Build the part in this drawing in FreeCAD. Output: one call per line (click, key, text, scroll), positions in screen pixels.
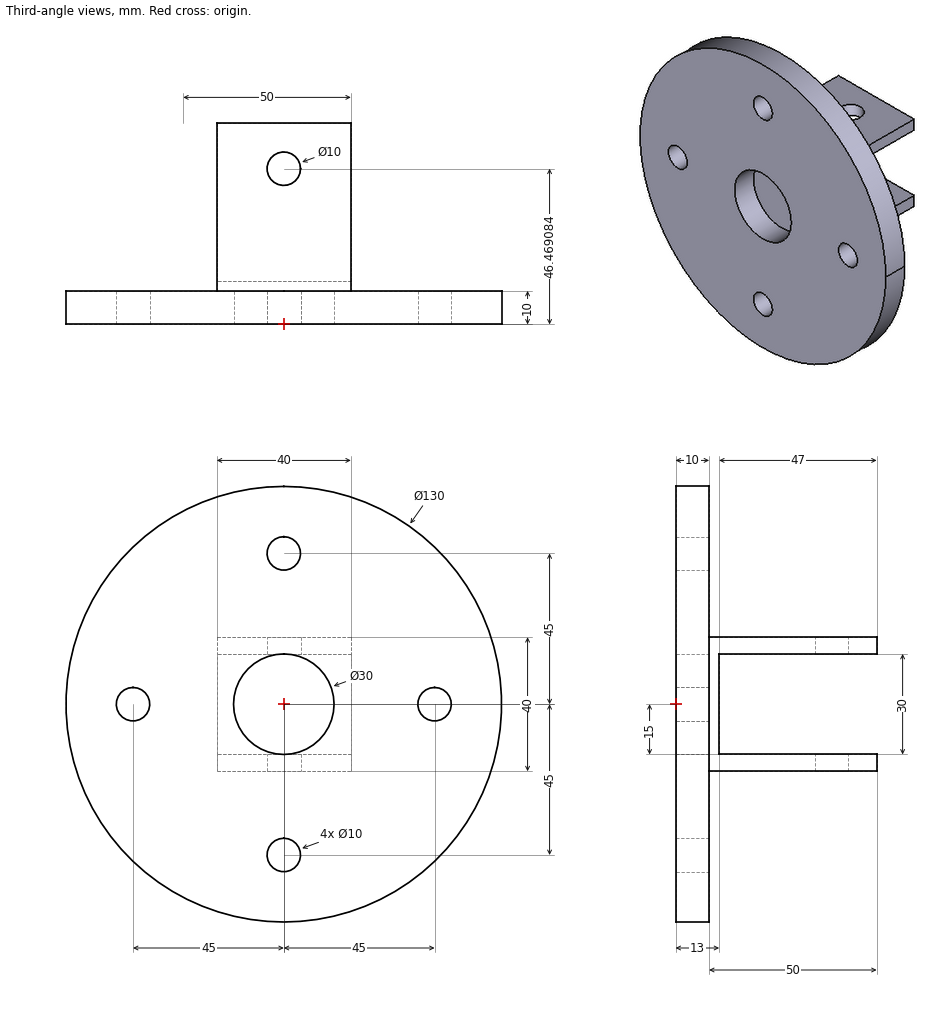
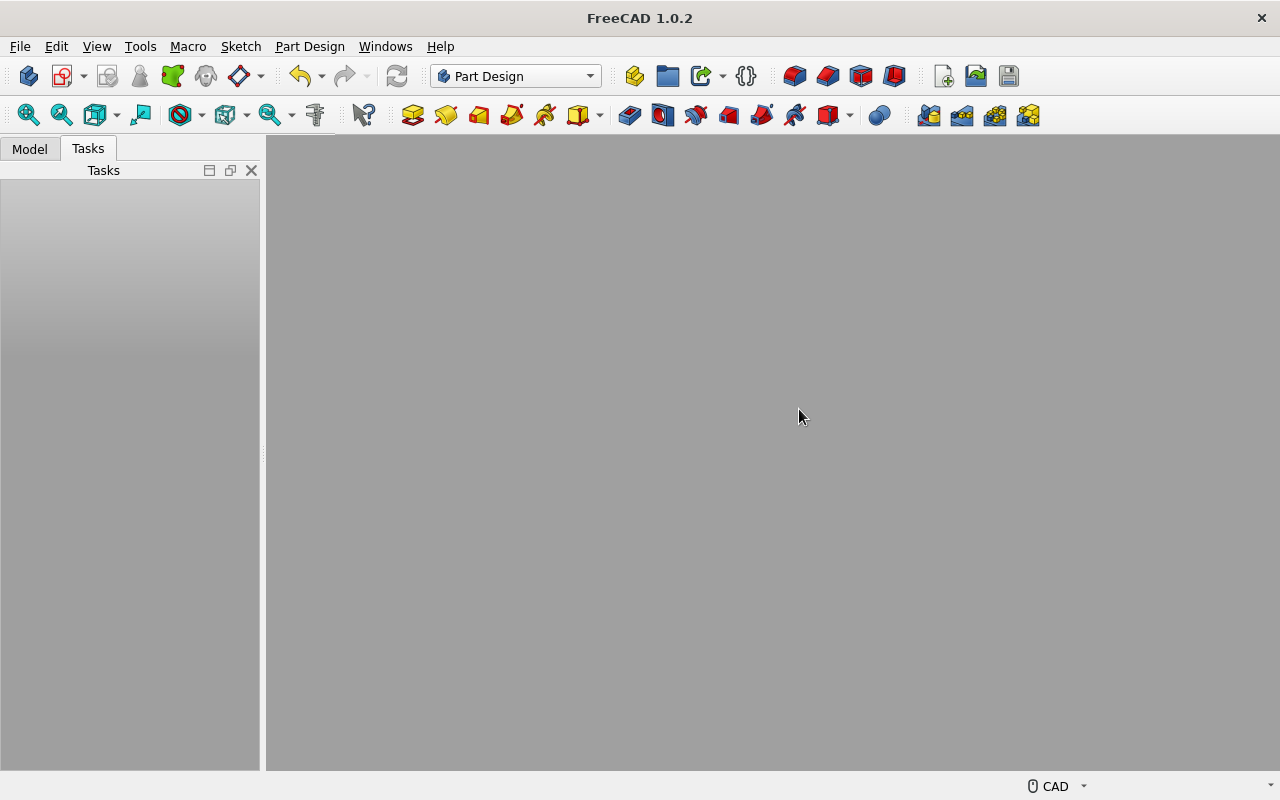
click(943, 76)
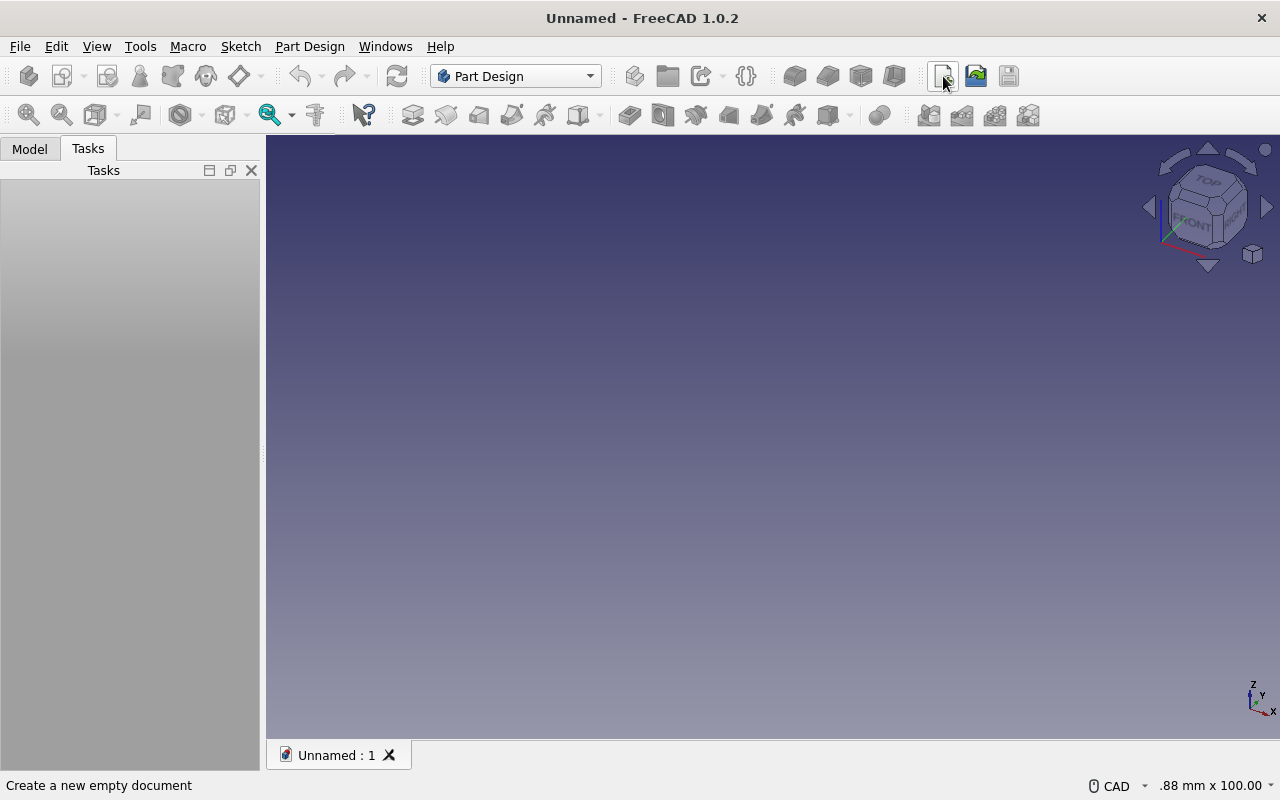
click(62, 76)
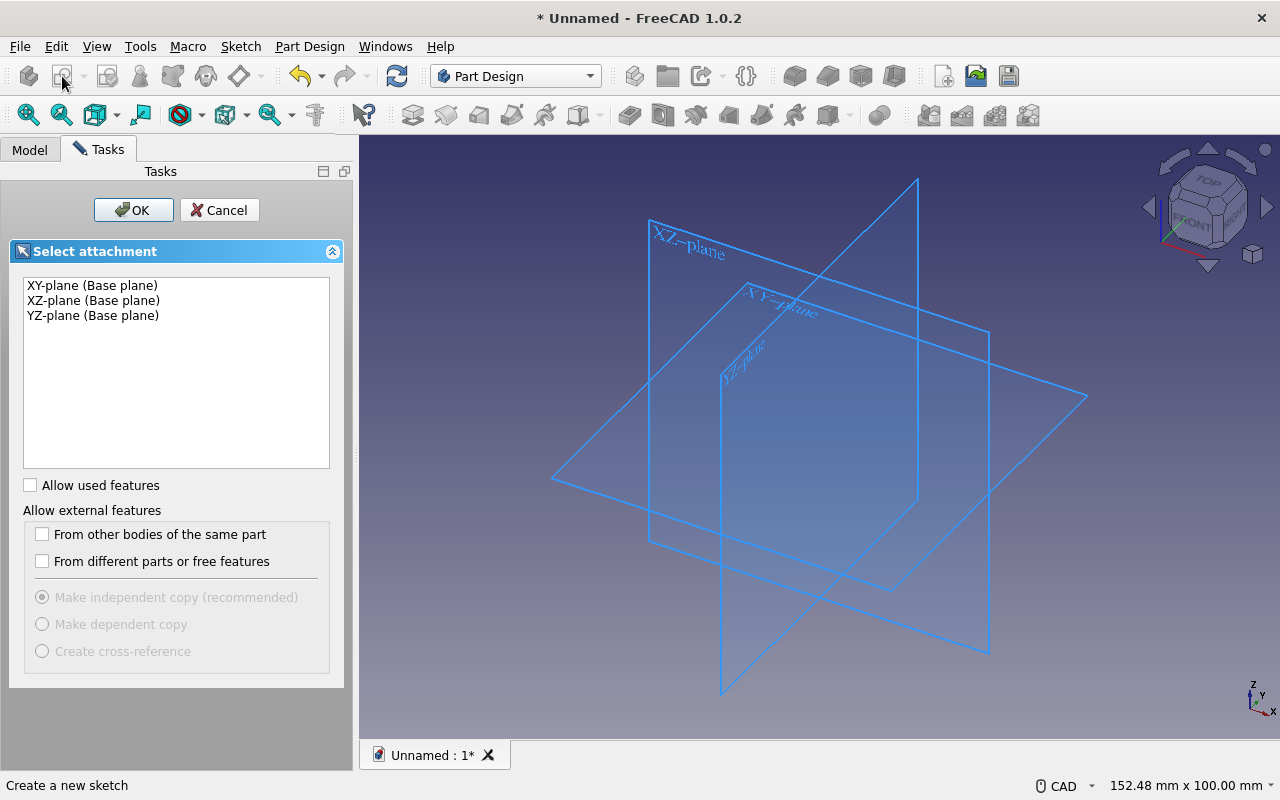
click(84, 300)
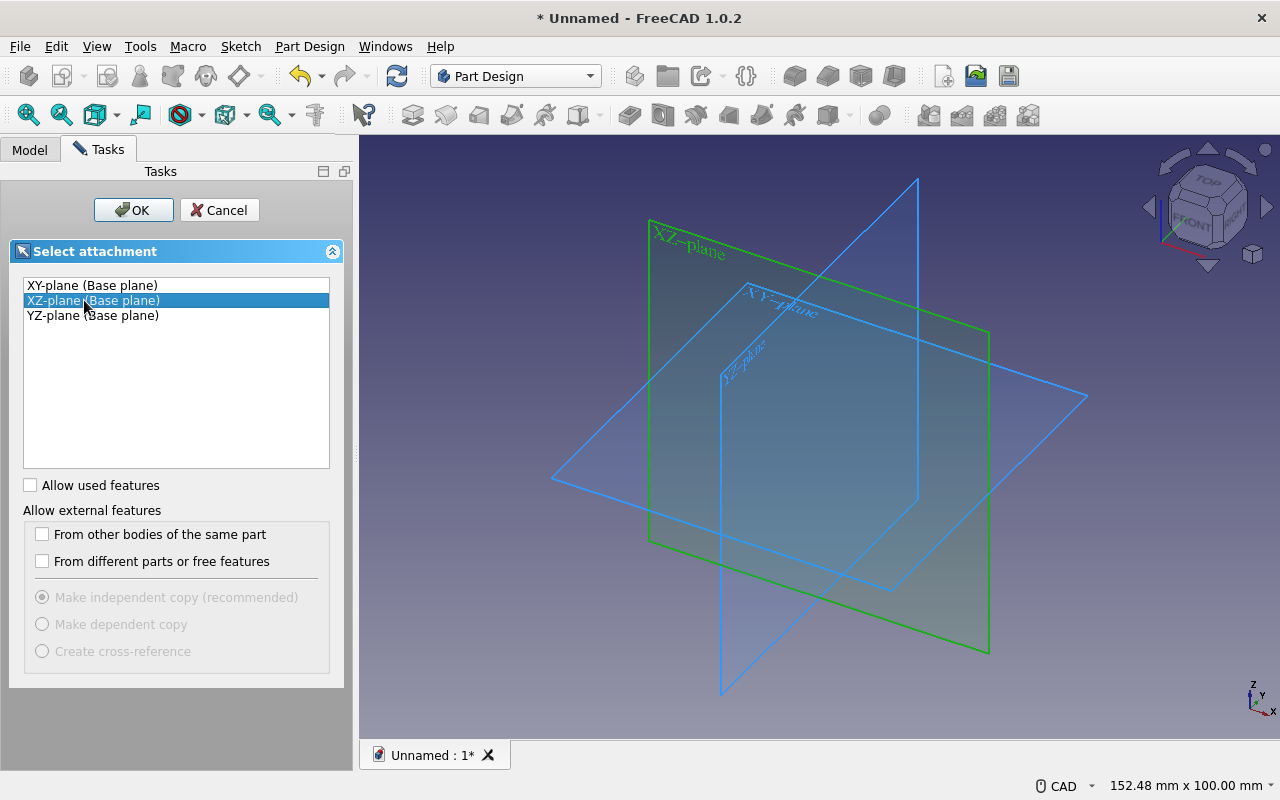
click(134, 210)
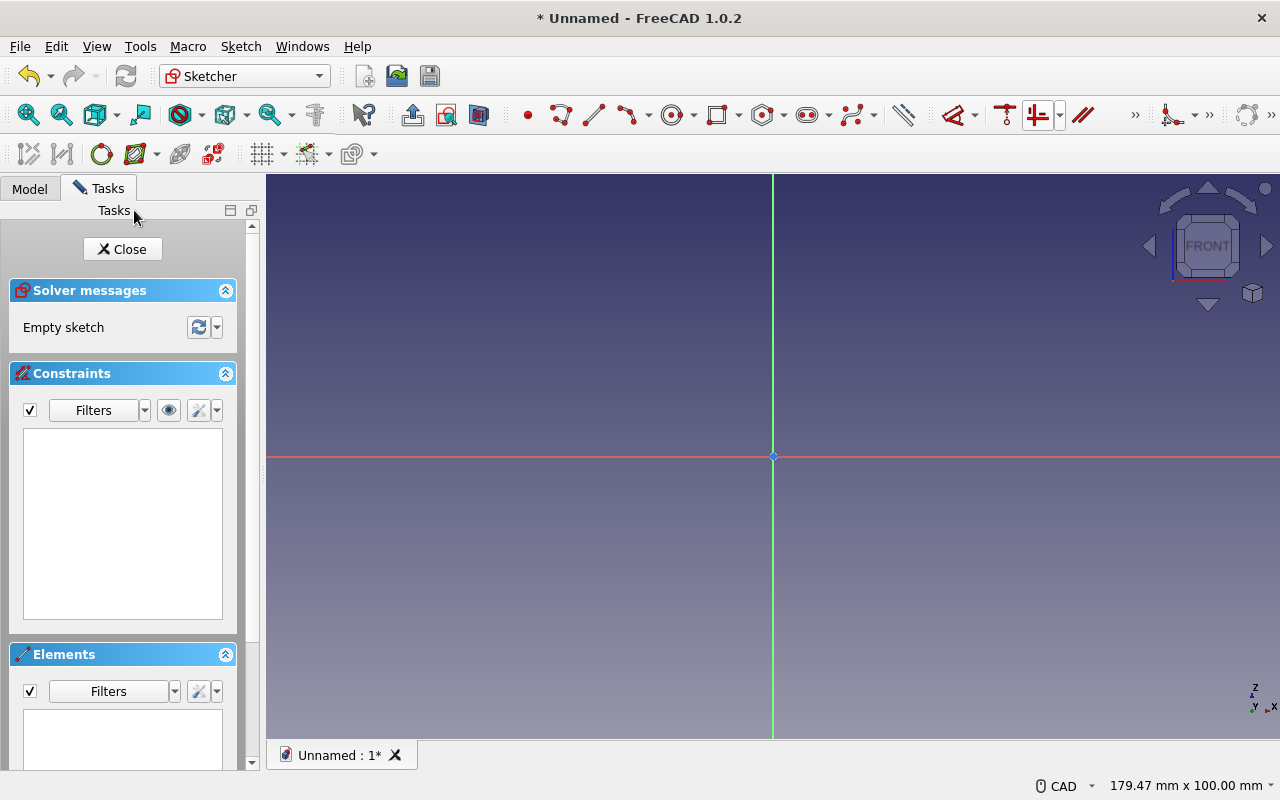
scroll(649, 456, down, 4)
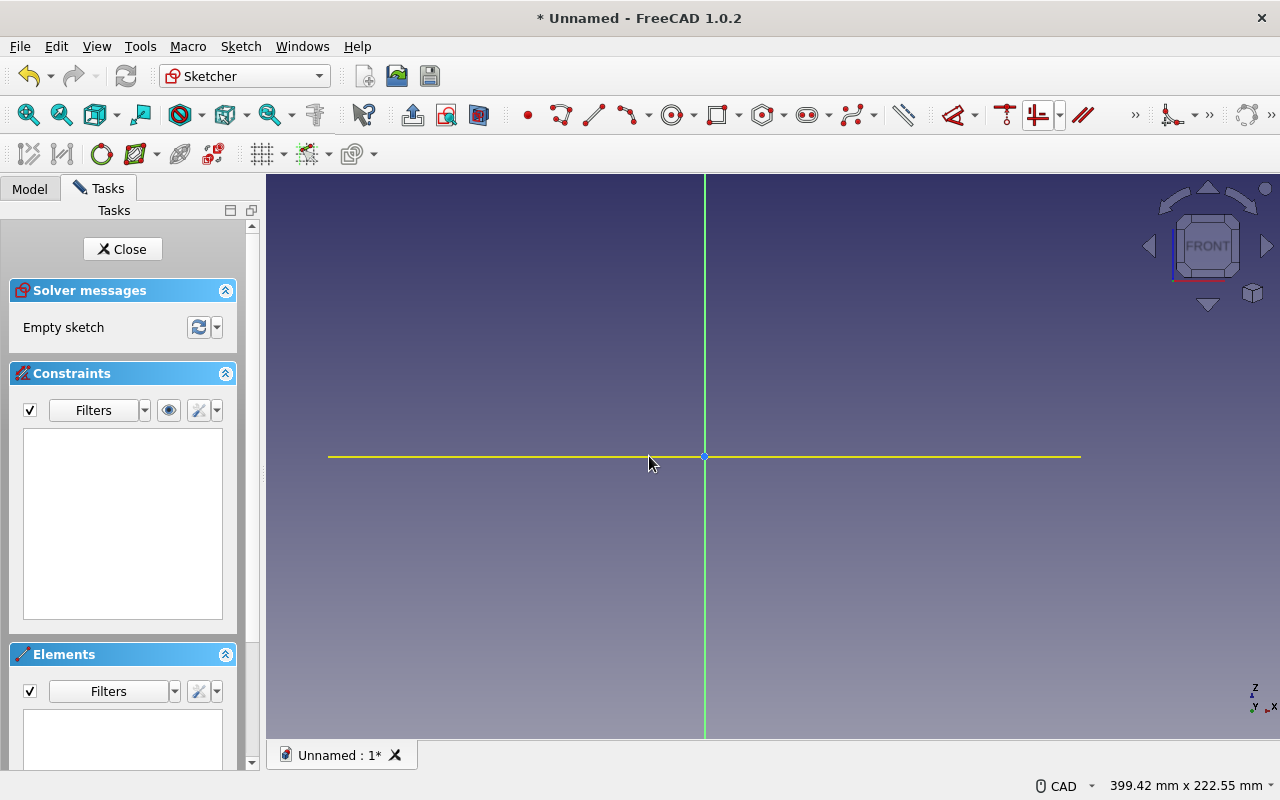
key(g)
key(c)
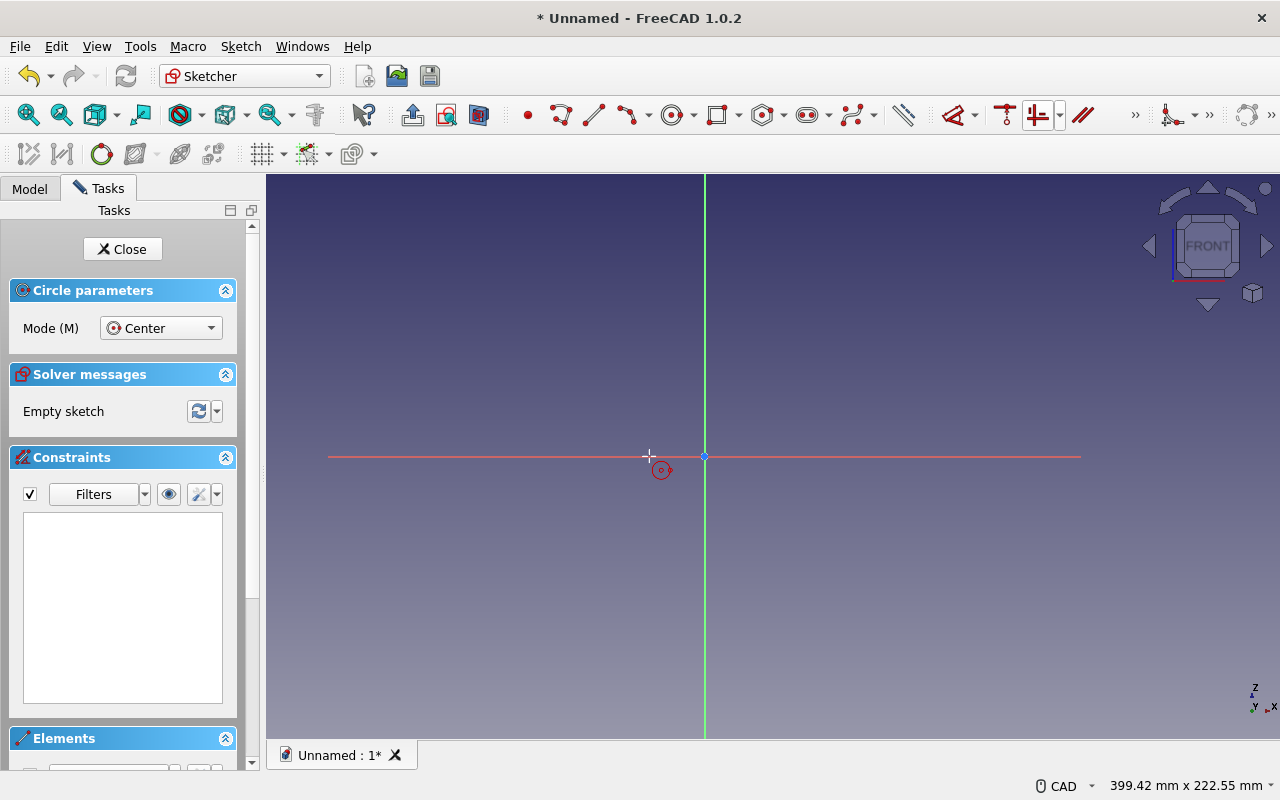
click(705, 456)
move(822, 340)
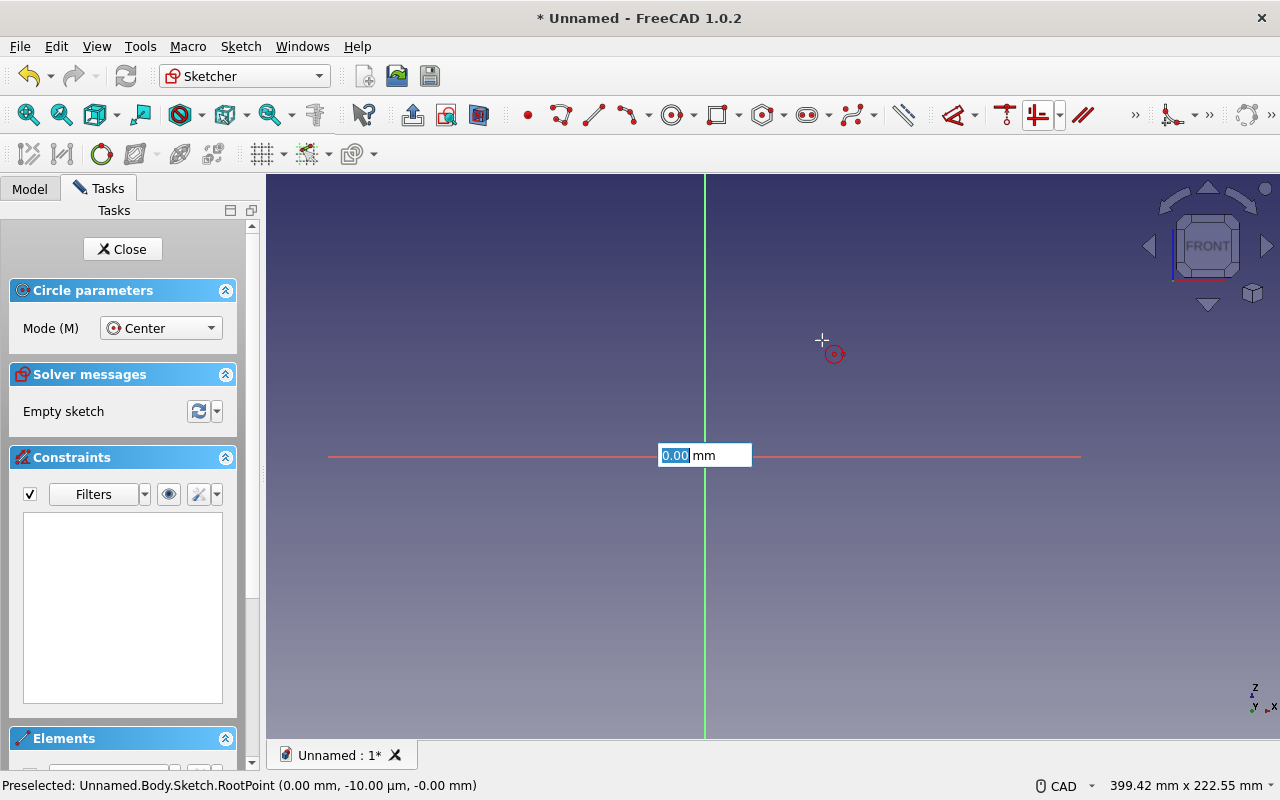
text(130)
key(Return)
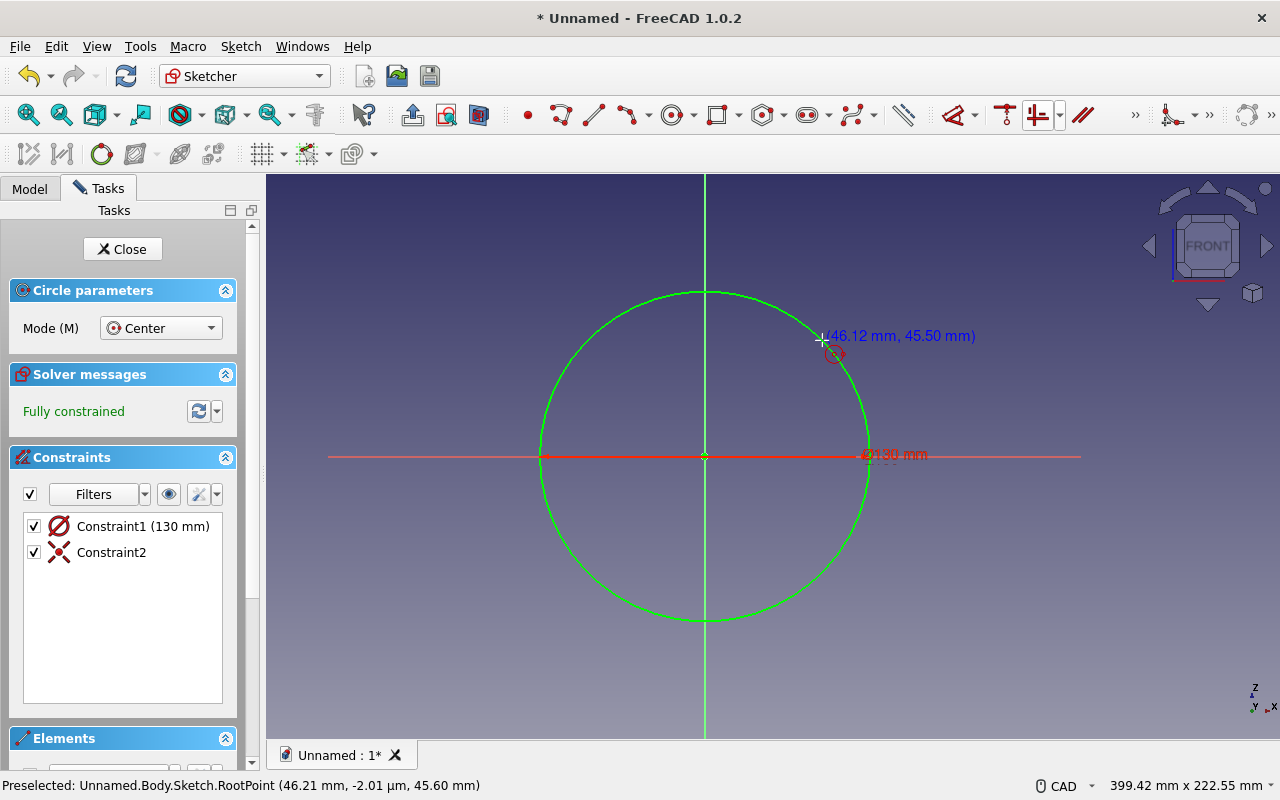
click(705, 456)
move(732, 430)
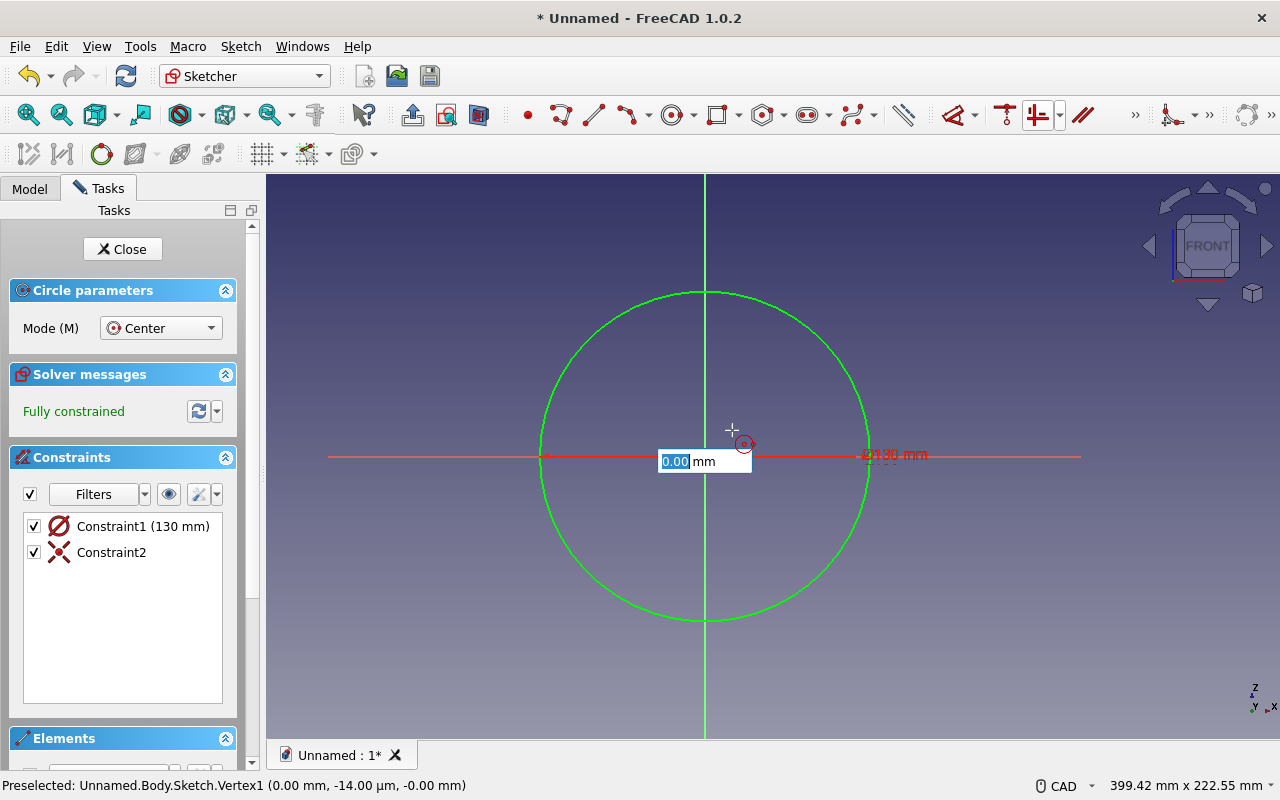
text(30)
key(Return)
key(Escape)